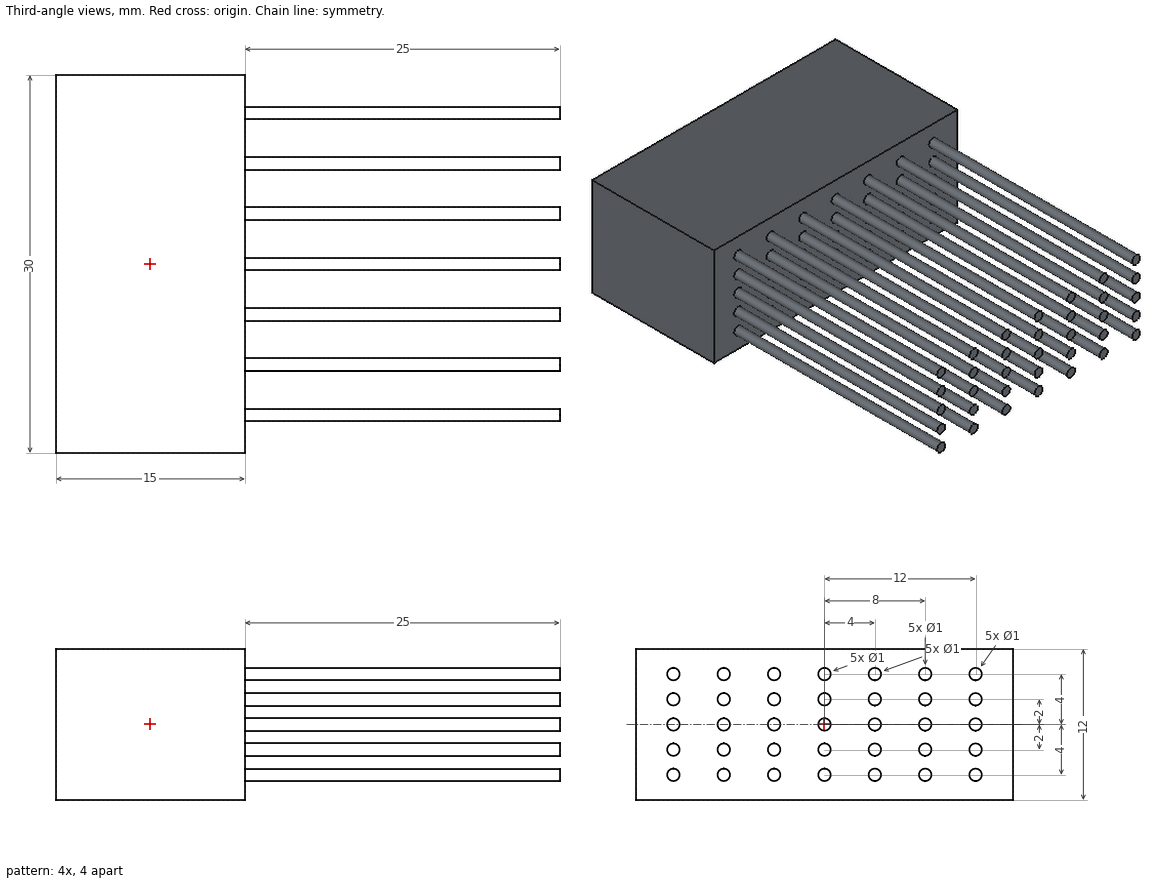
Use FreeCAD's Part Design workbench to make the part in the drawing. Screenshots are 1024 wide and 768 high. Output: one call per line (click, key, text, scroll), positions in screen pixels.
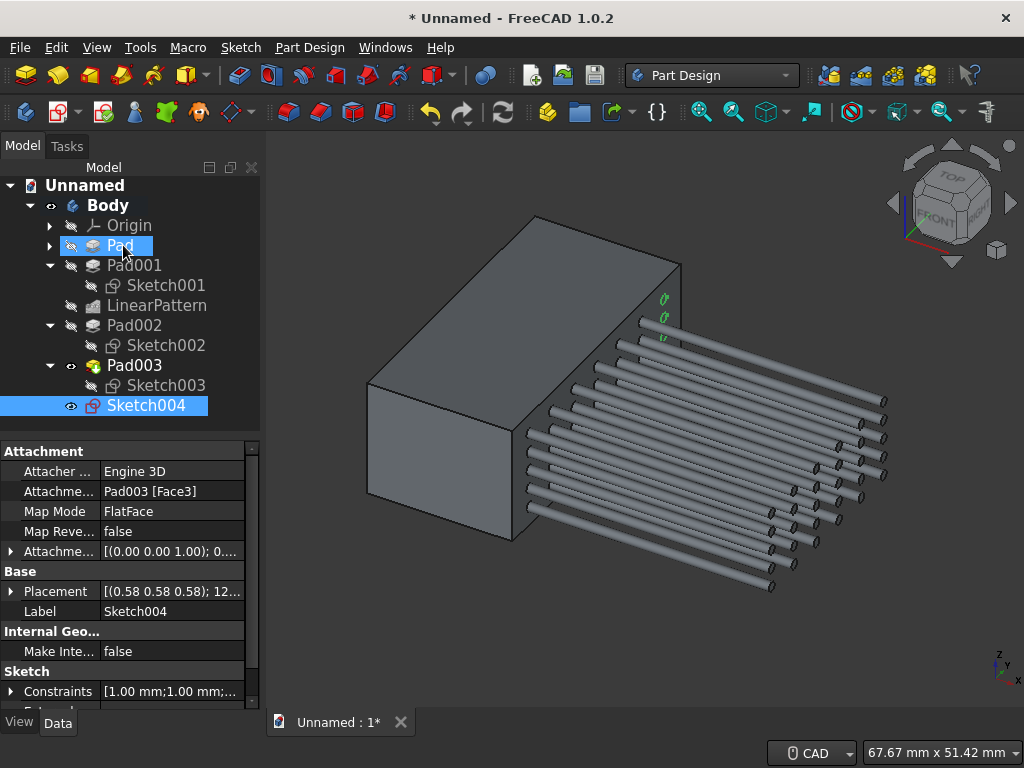
click(26, 76)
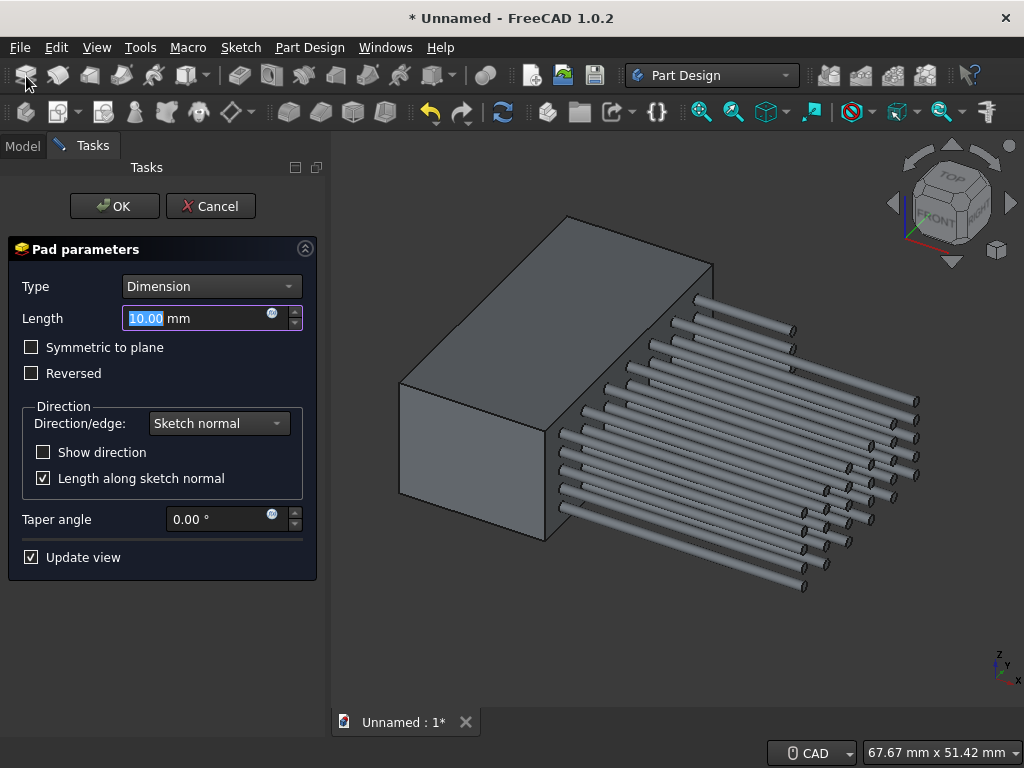
text(25)
key(Tab)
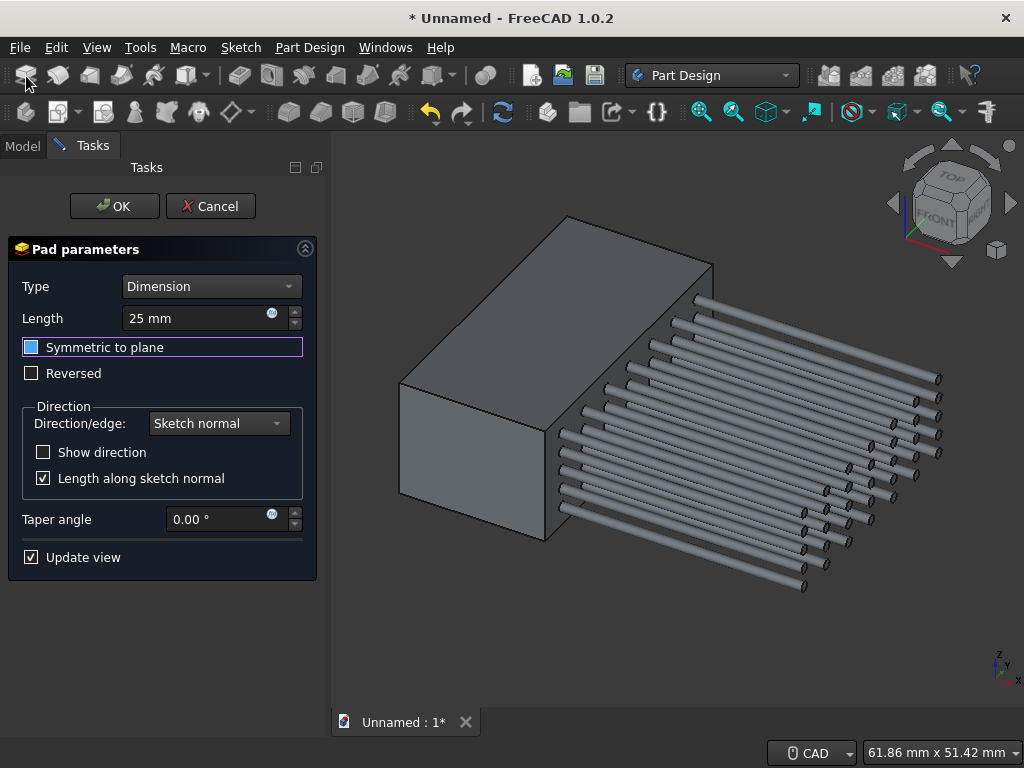
click(115, 206)